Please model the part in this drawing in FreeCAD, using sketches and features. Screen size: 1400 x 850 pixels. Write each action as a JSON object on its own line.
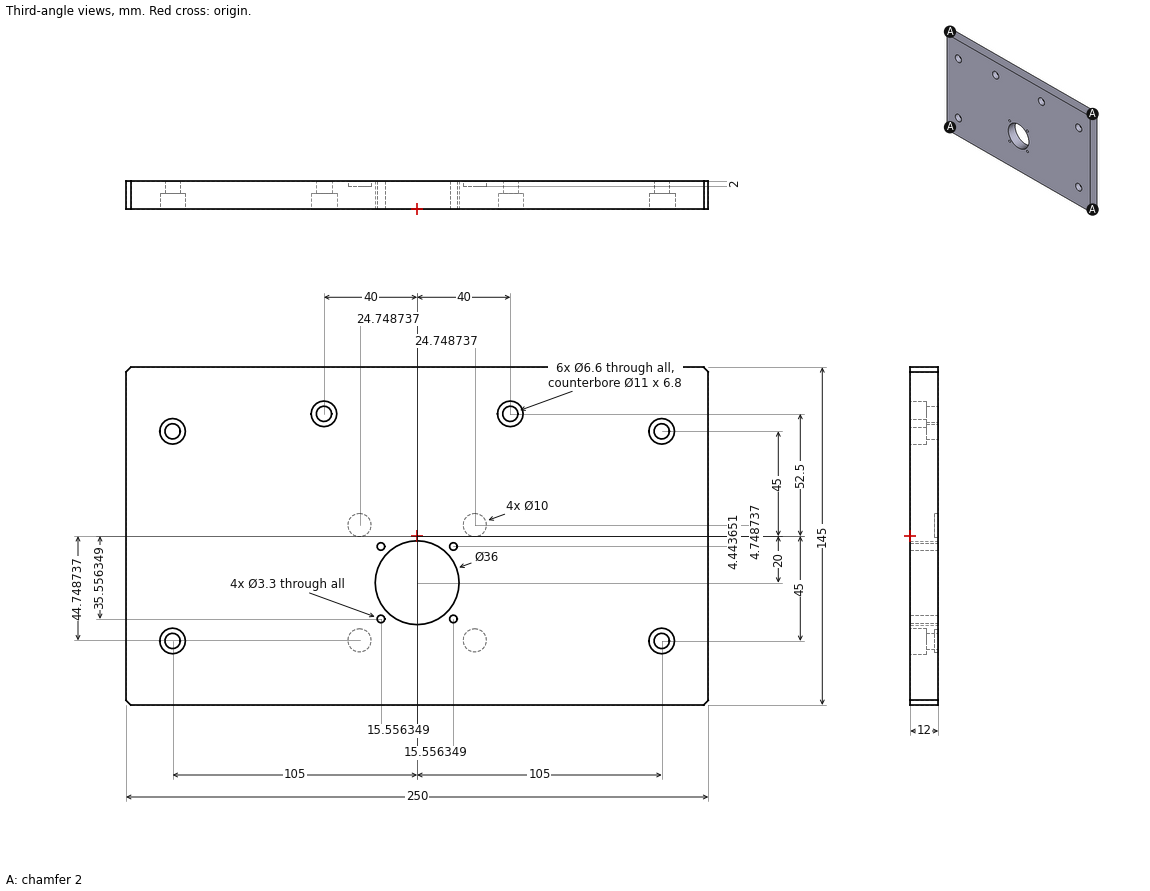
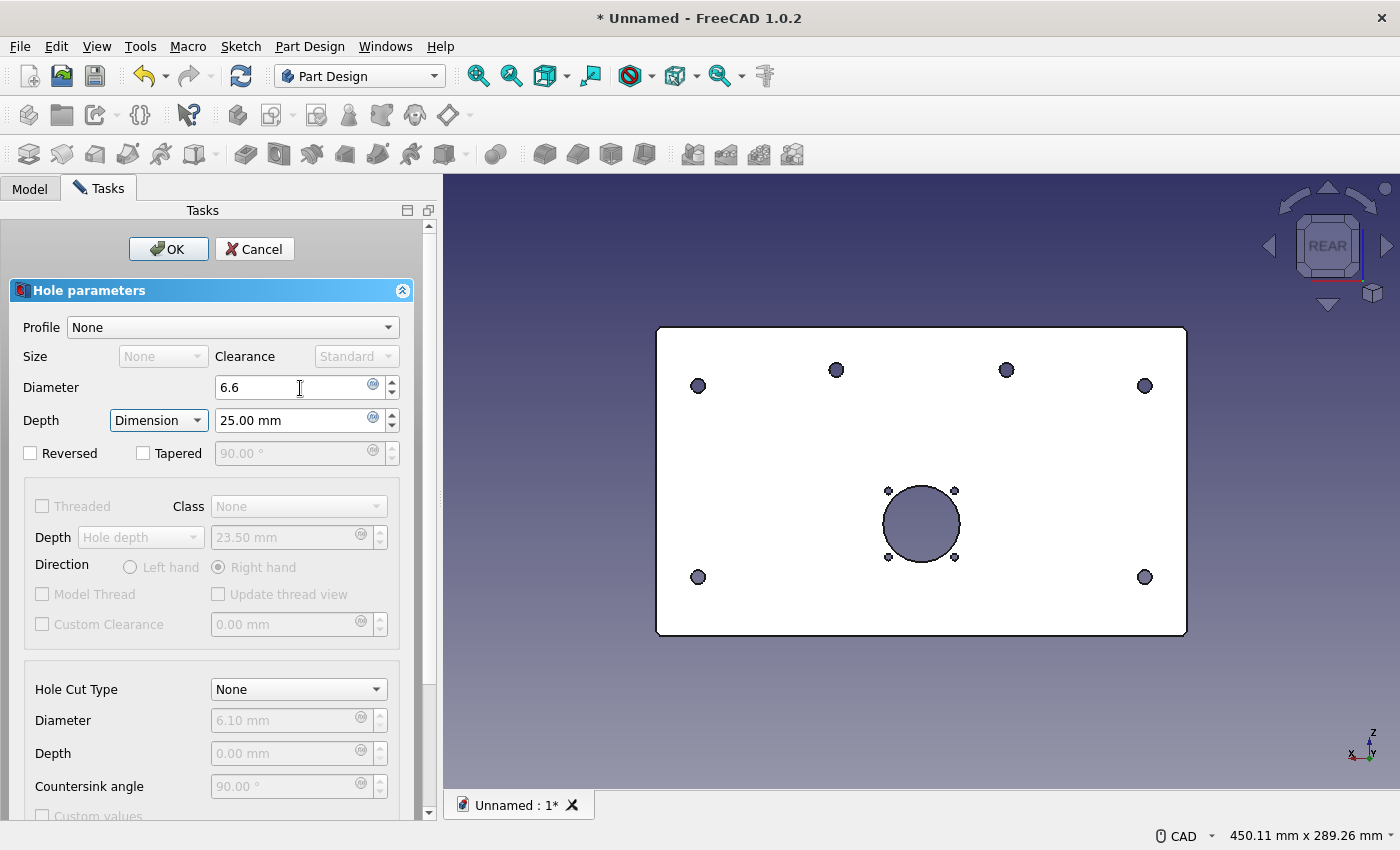
{"action": "left_click", "coordinate": [160, 420]}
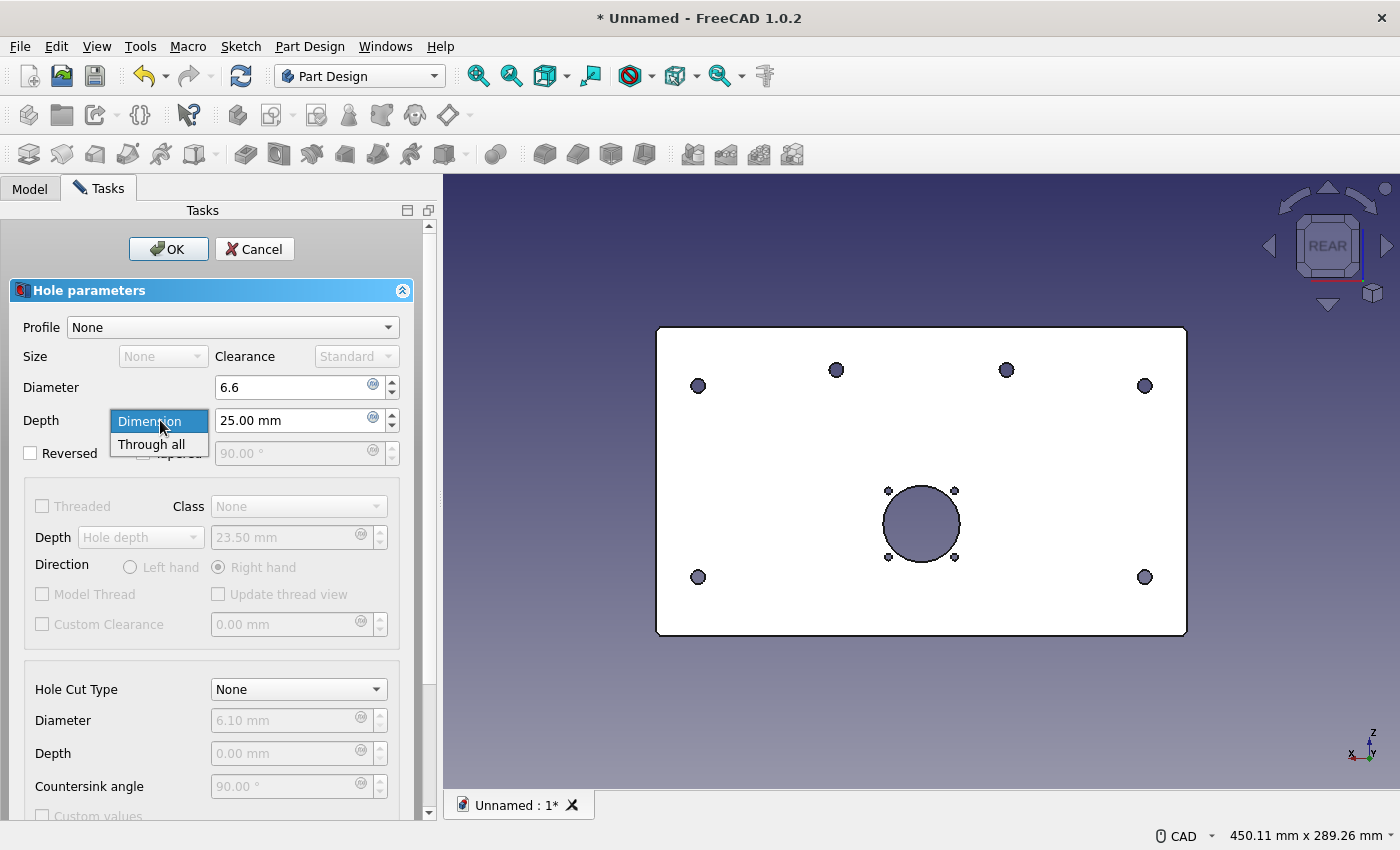
{"action": "left_click", "coordinate": [158, 444]}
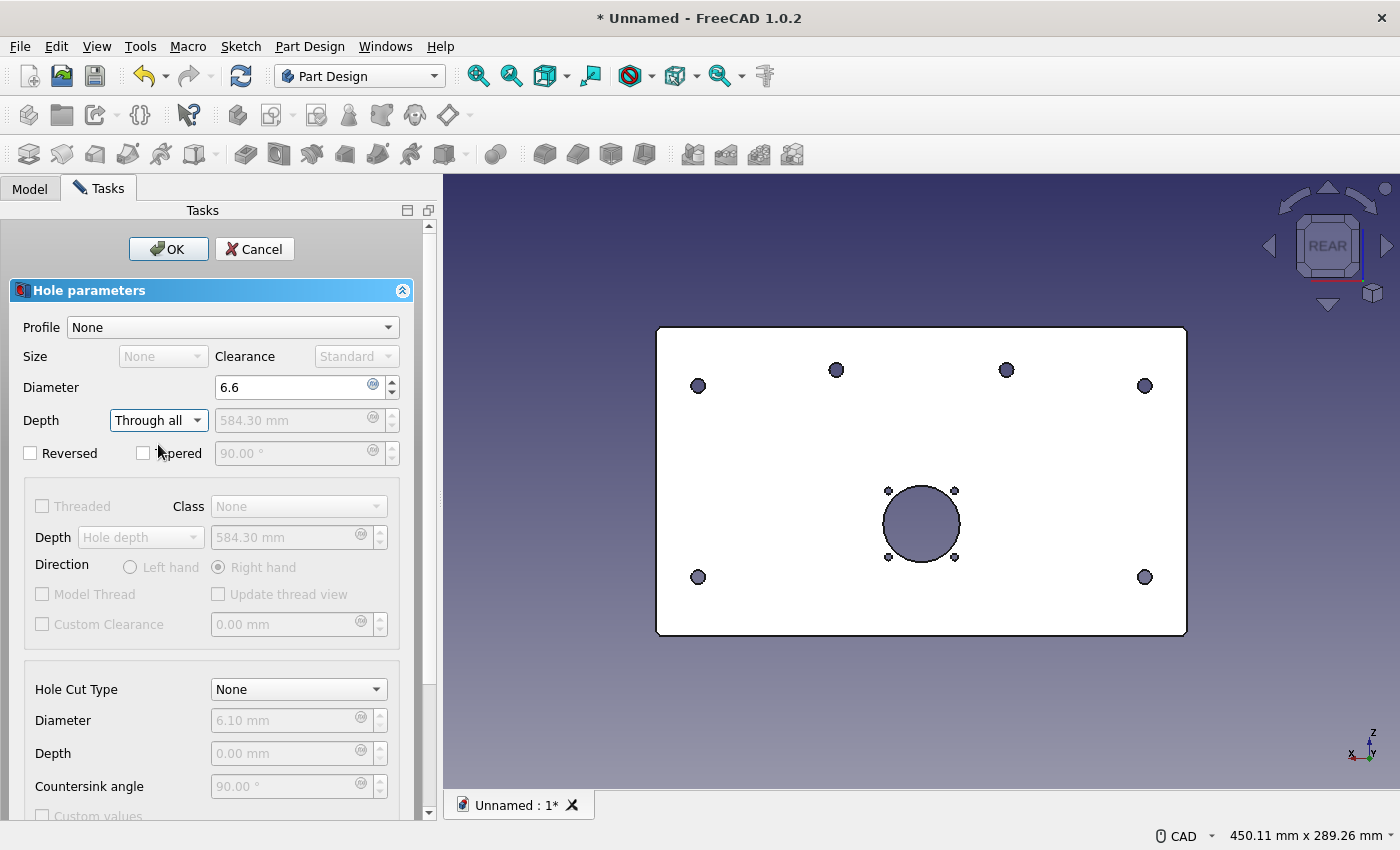
{"action": "left_click", "coordinate": [300, 690]}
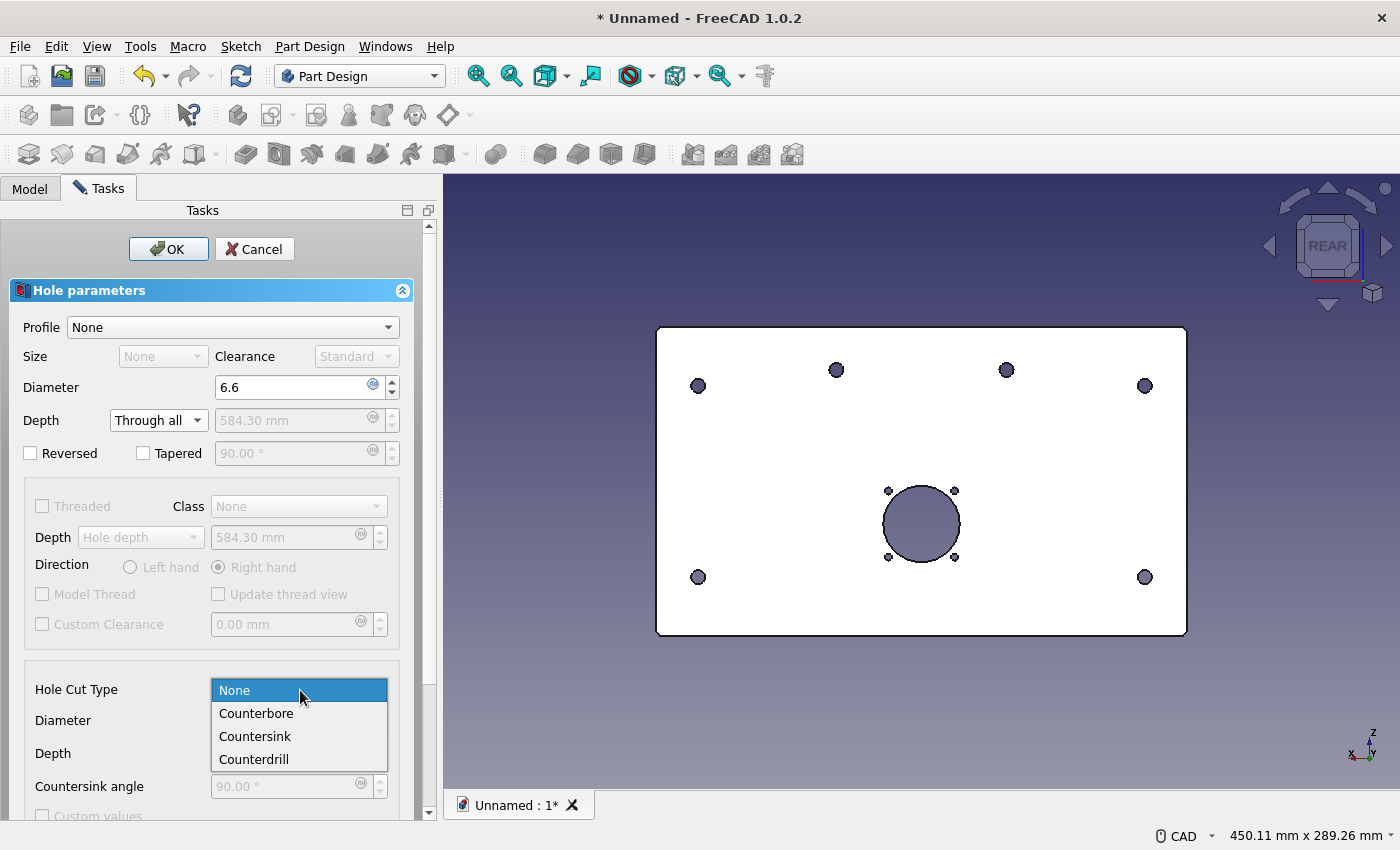
{"action": "left_click", "coordinate": [298, 714]}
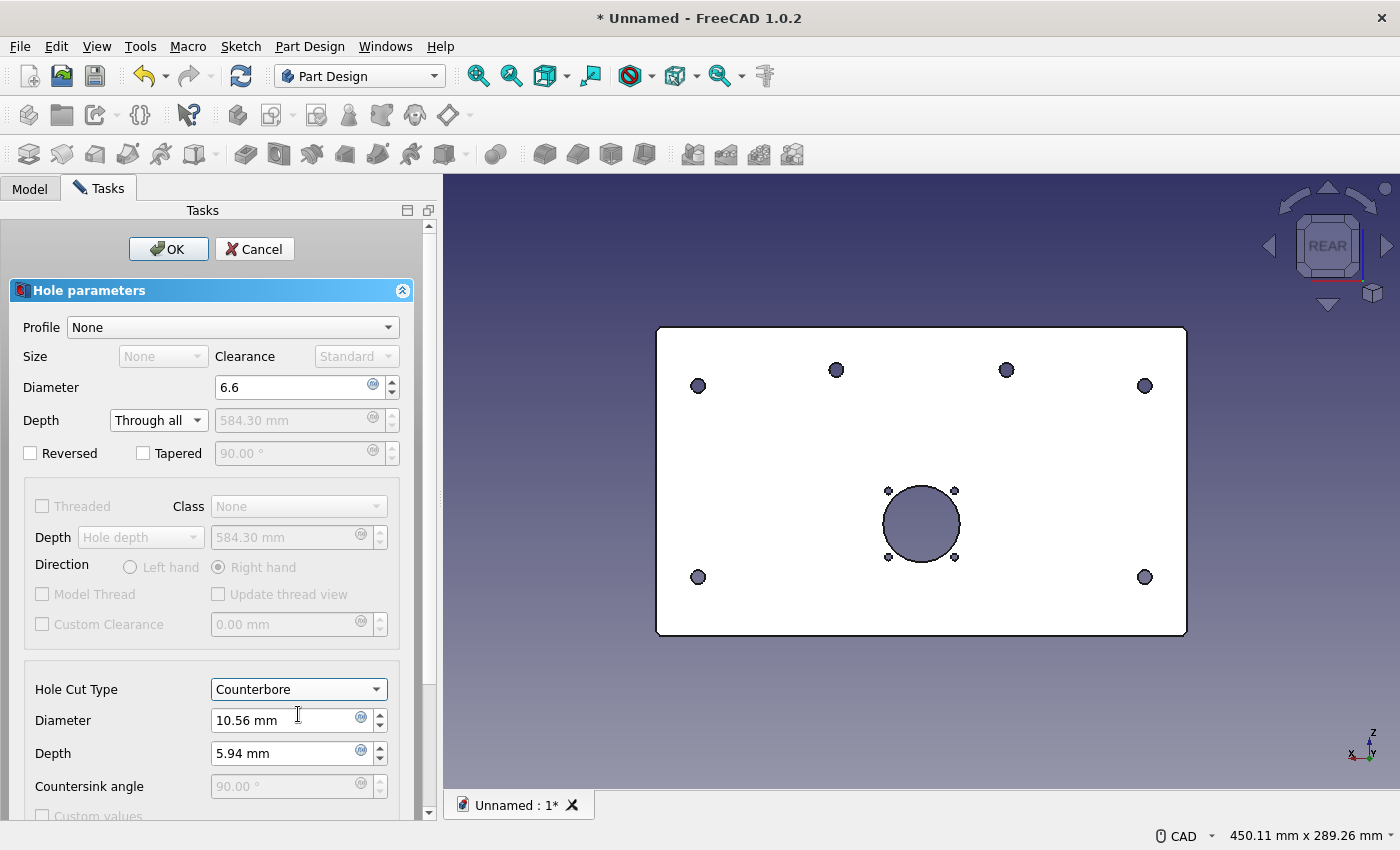
{"action": "triple_click", "coordinate": [292, 720]}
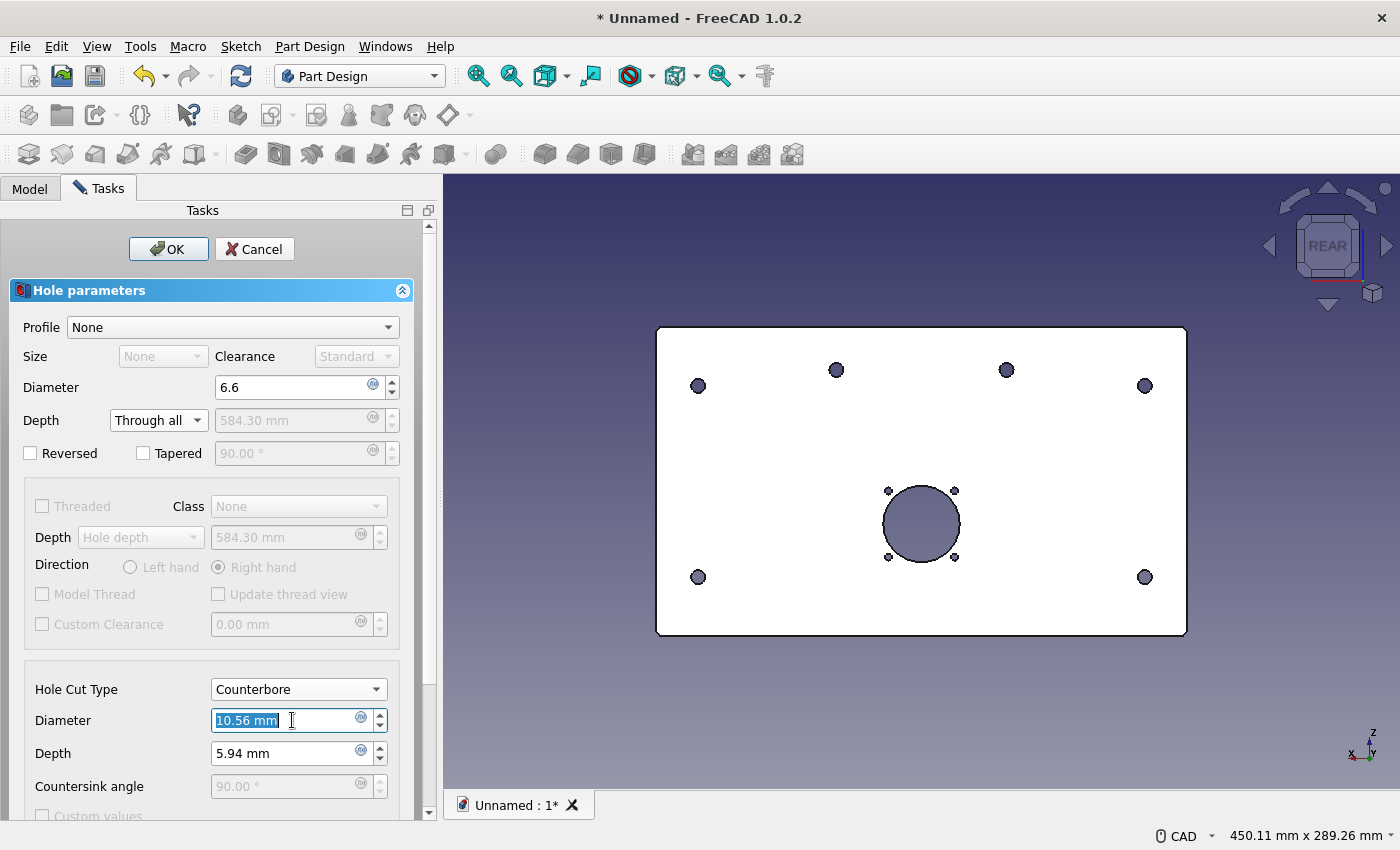
{"action": "type", "text": "11"}
{"action": "key", "text": "Tab"}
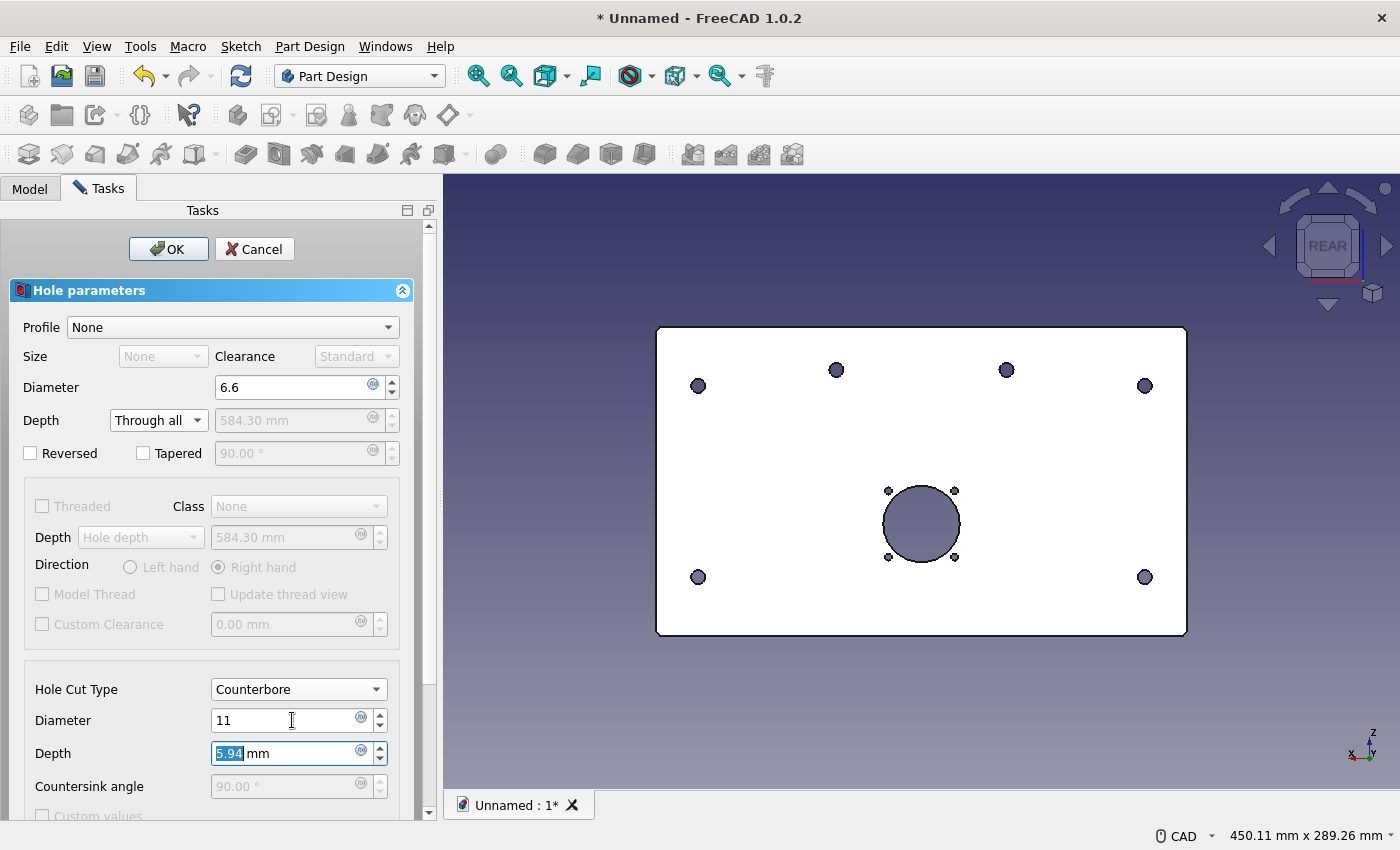
{"action": "type", "text": "6.8"}
{"action": "key", "text": "Tab"}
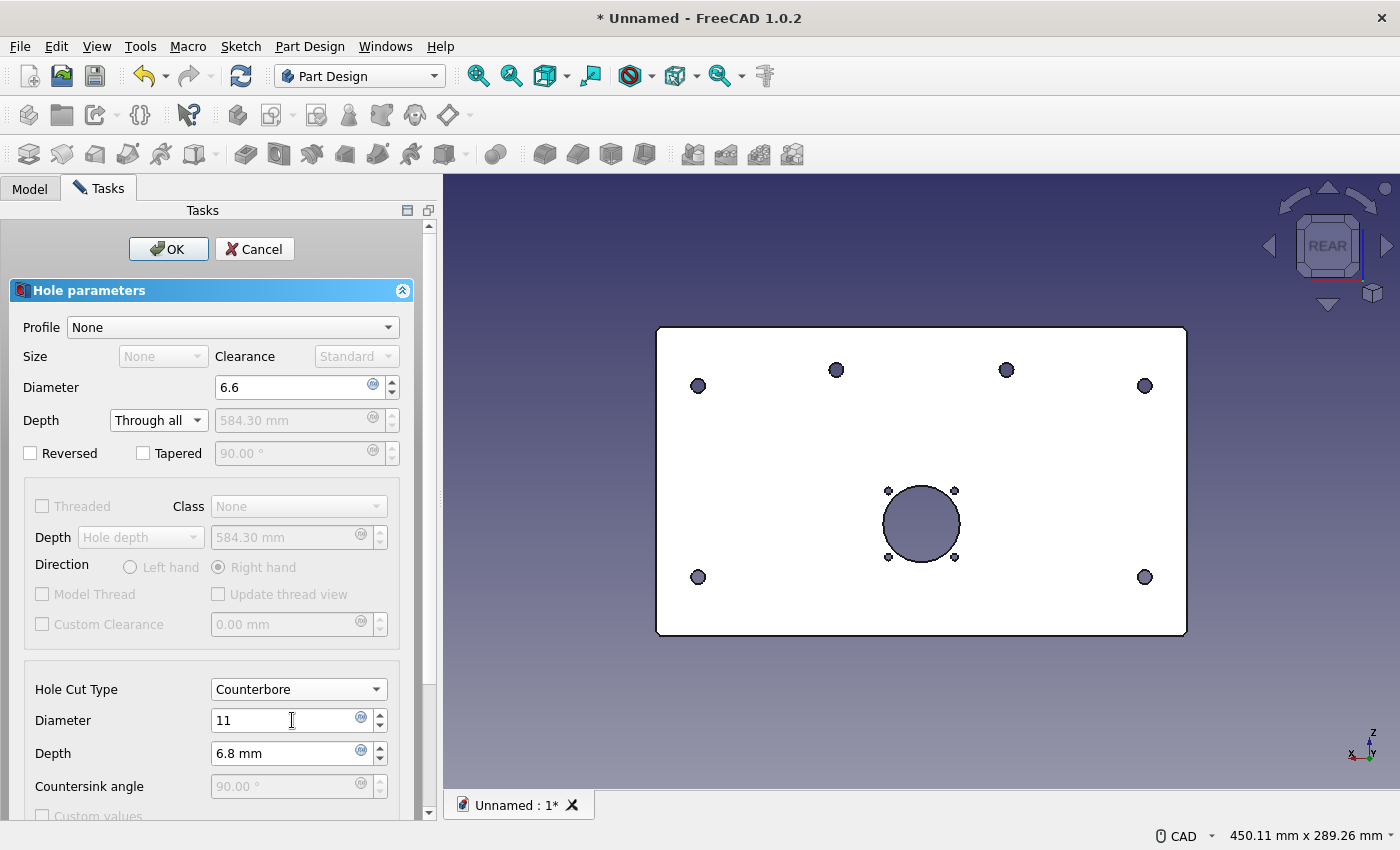
{"action": "left_click", "coordinate": [169, 249]}